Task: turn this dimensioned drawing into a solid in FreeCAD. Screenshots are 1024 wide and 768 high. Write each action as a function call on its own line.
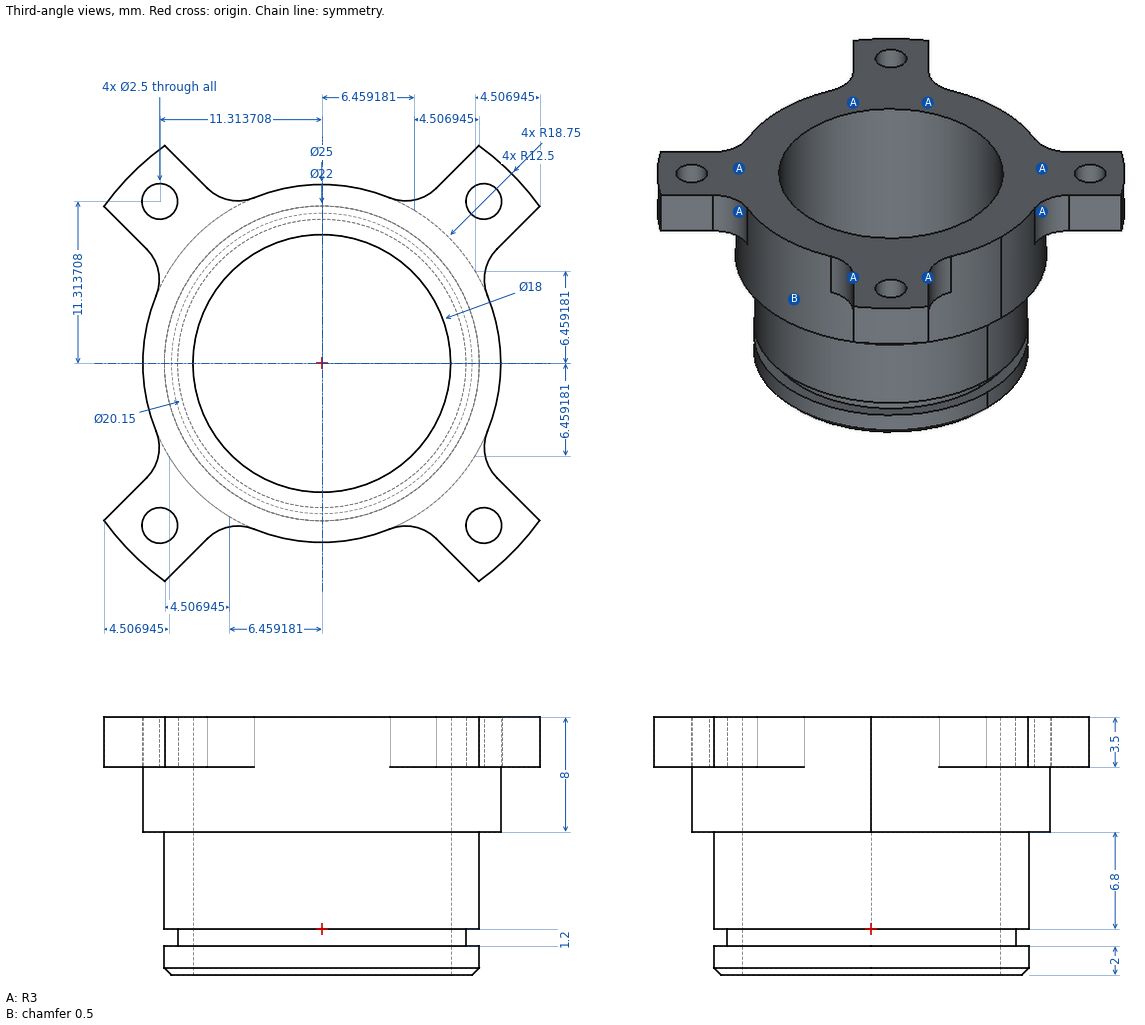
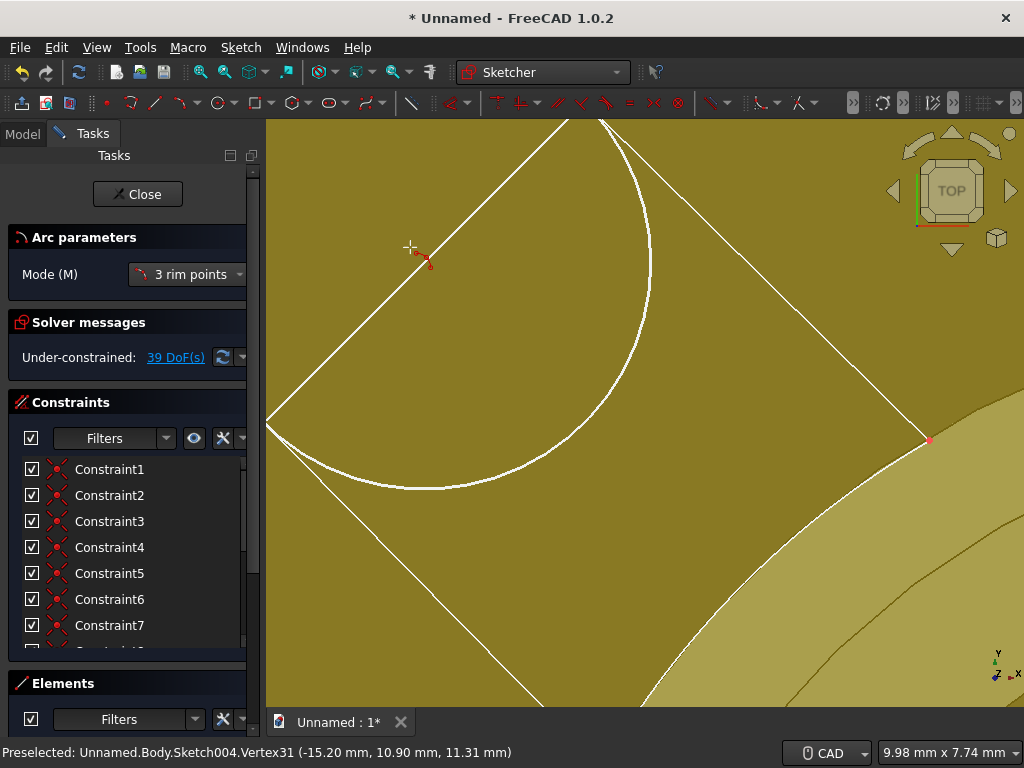
click(411, 243)
key(Escape)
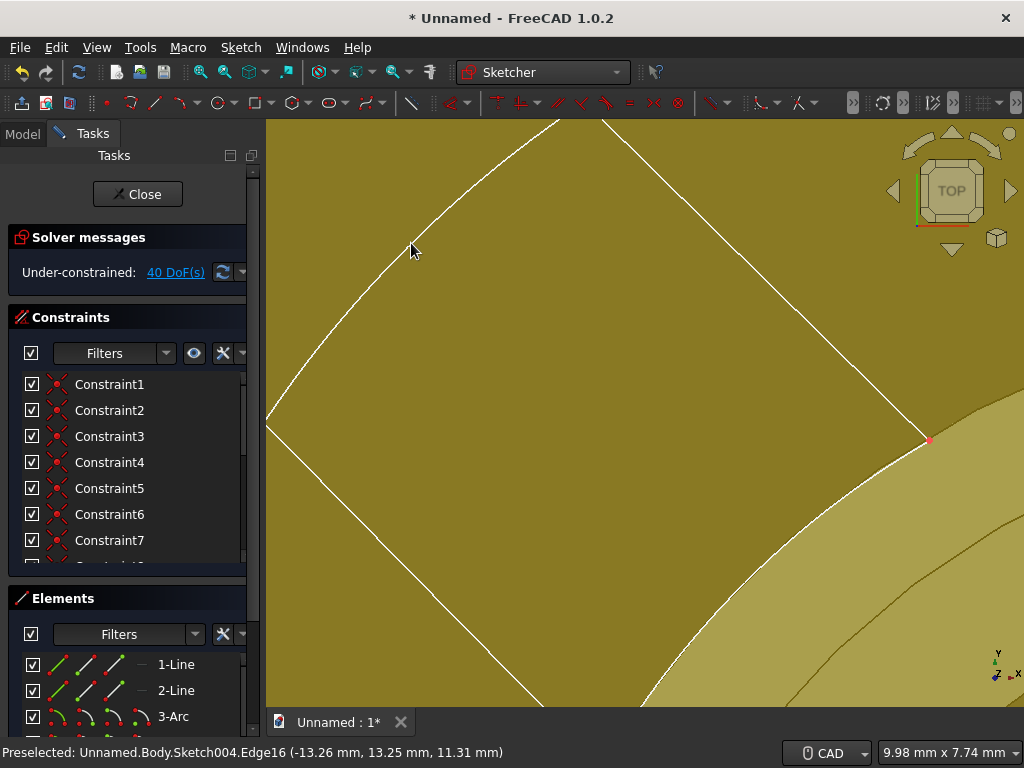
scroll(410, 247, down, 9)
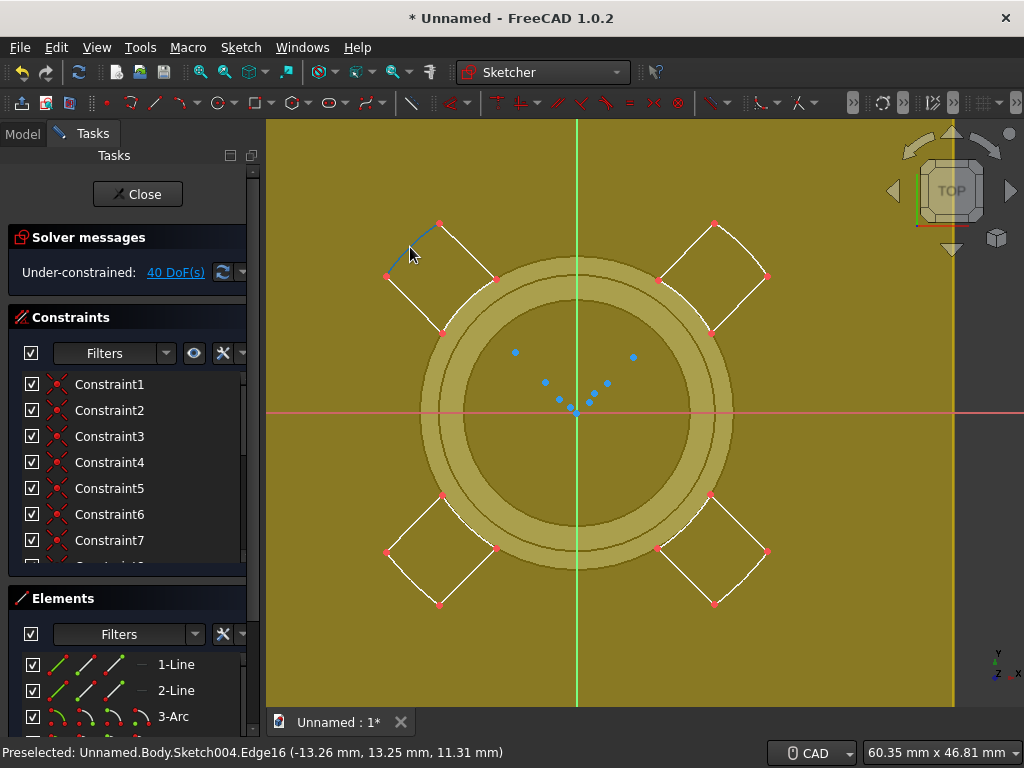
click(699, 314)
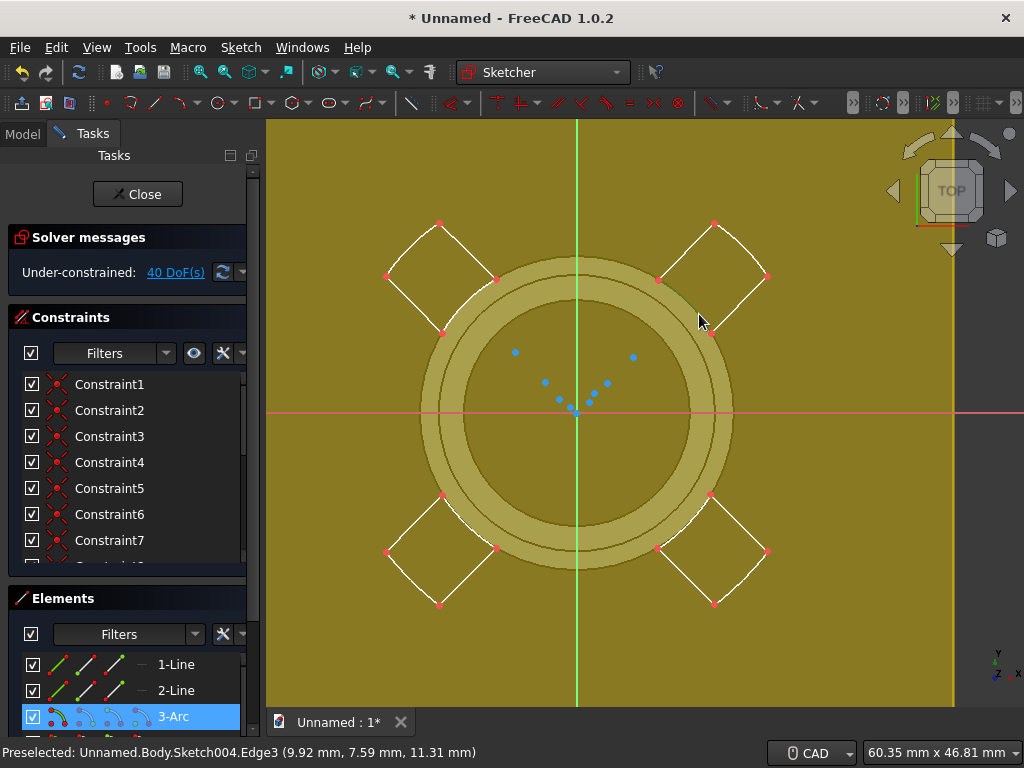
click(754, 258)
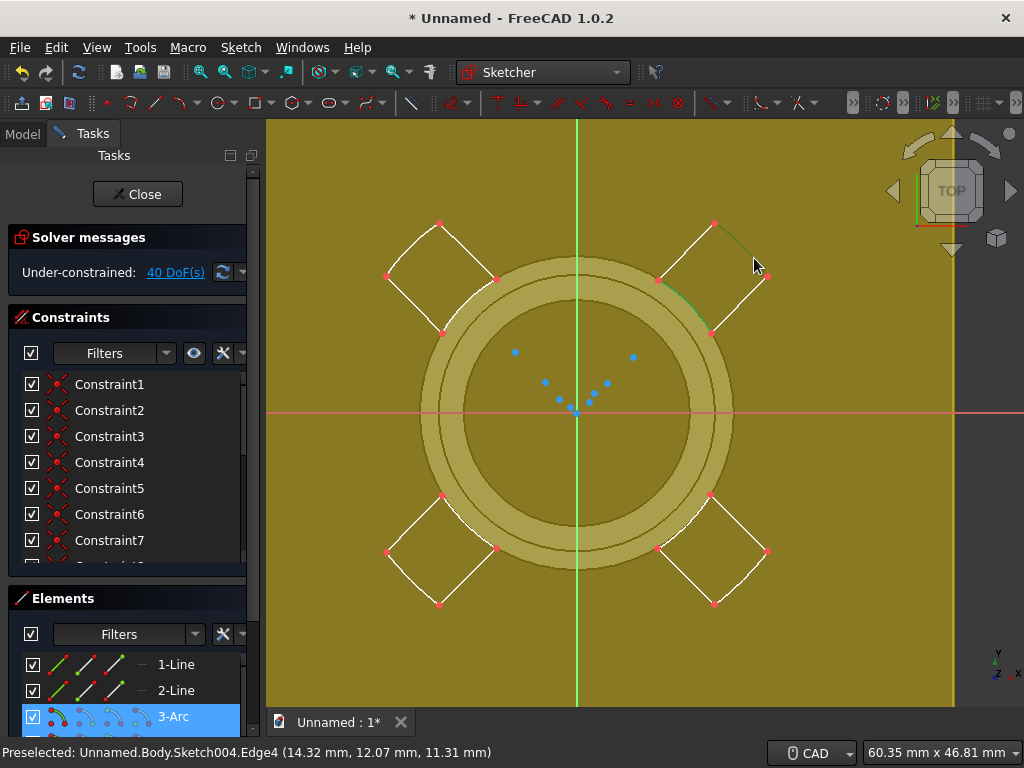
click(498, 104)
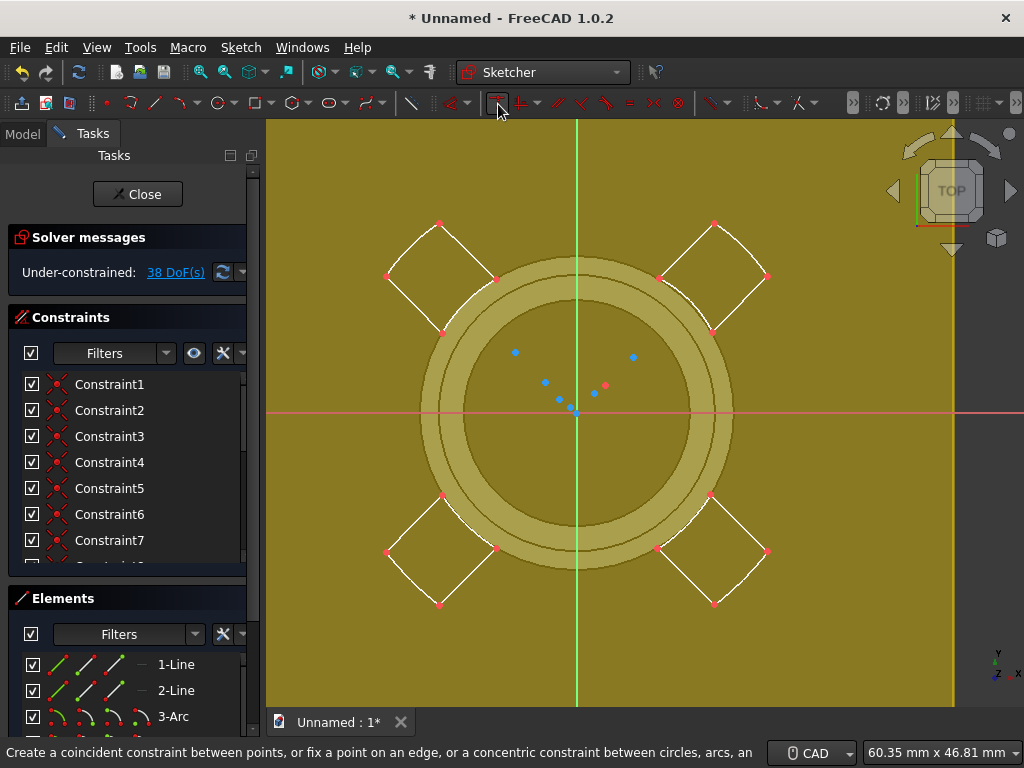
click(700, 313)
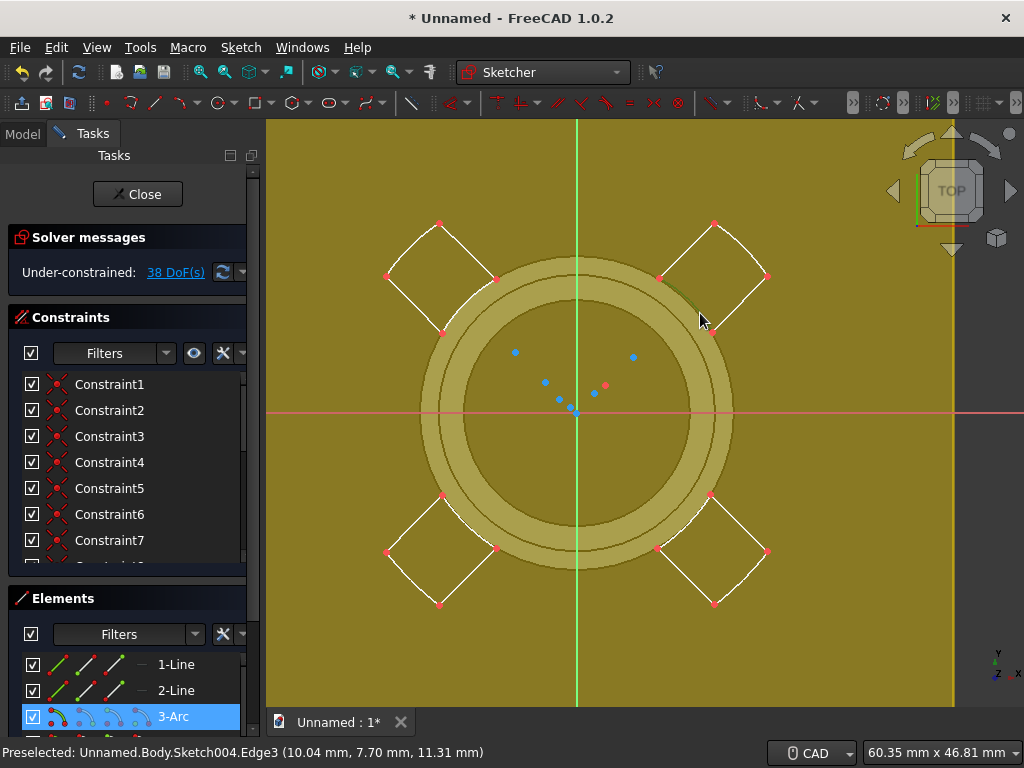
click(676, 535)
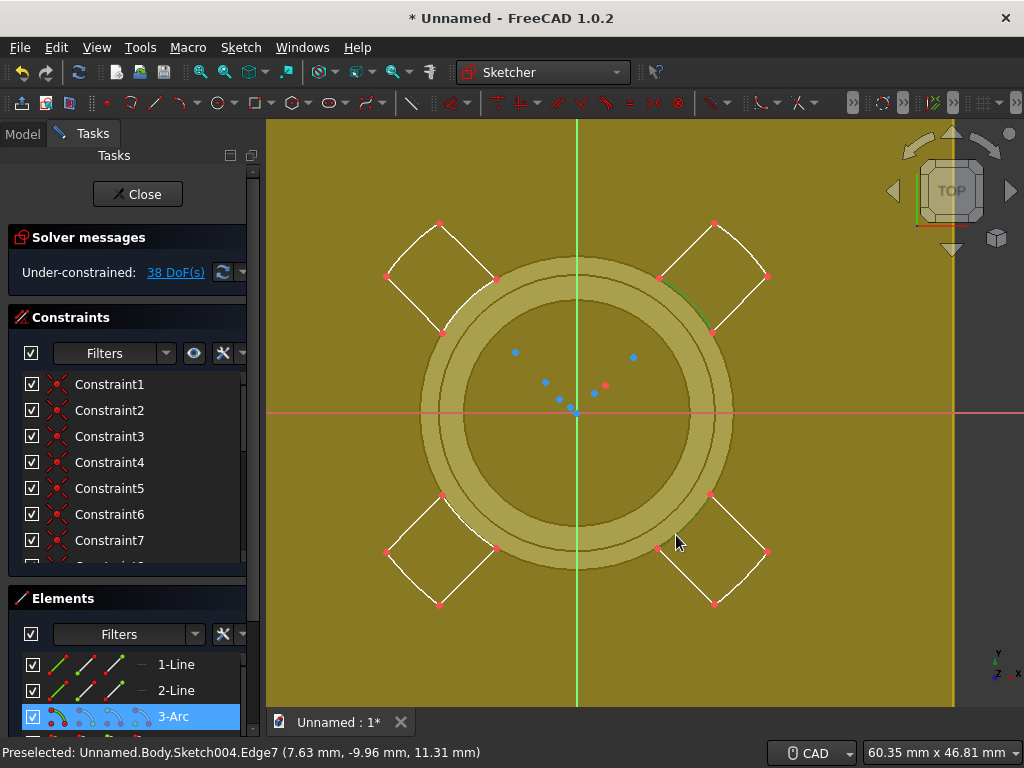
click(498, 104)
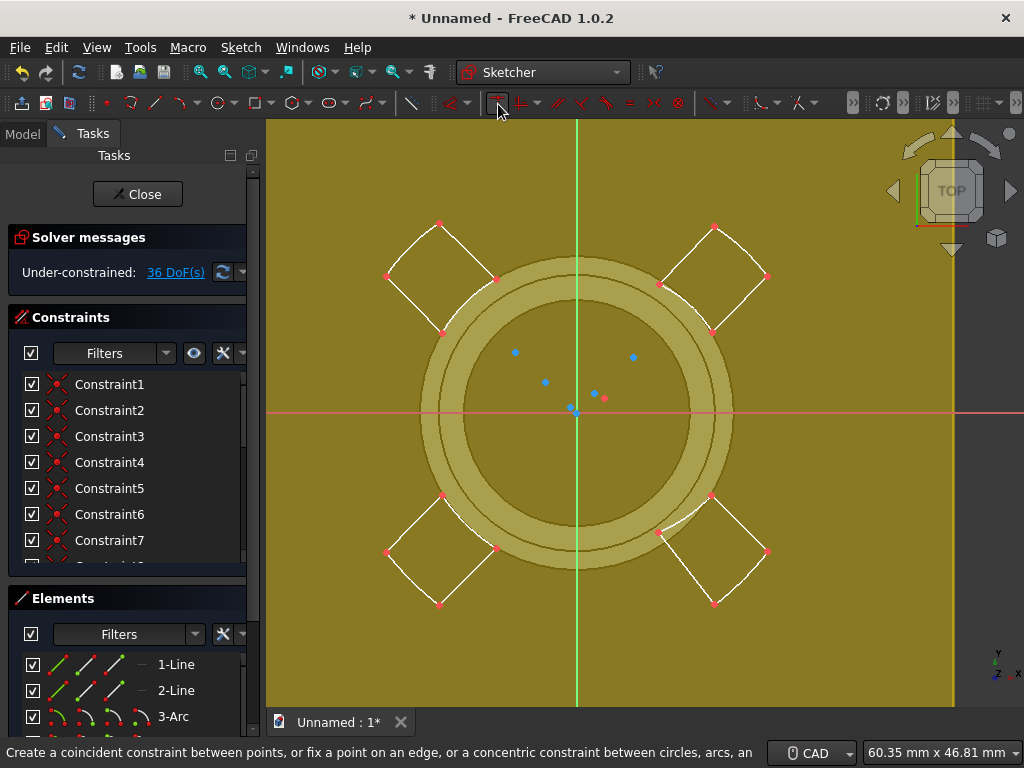
click(699, 315)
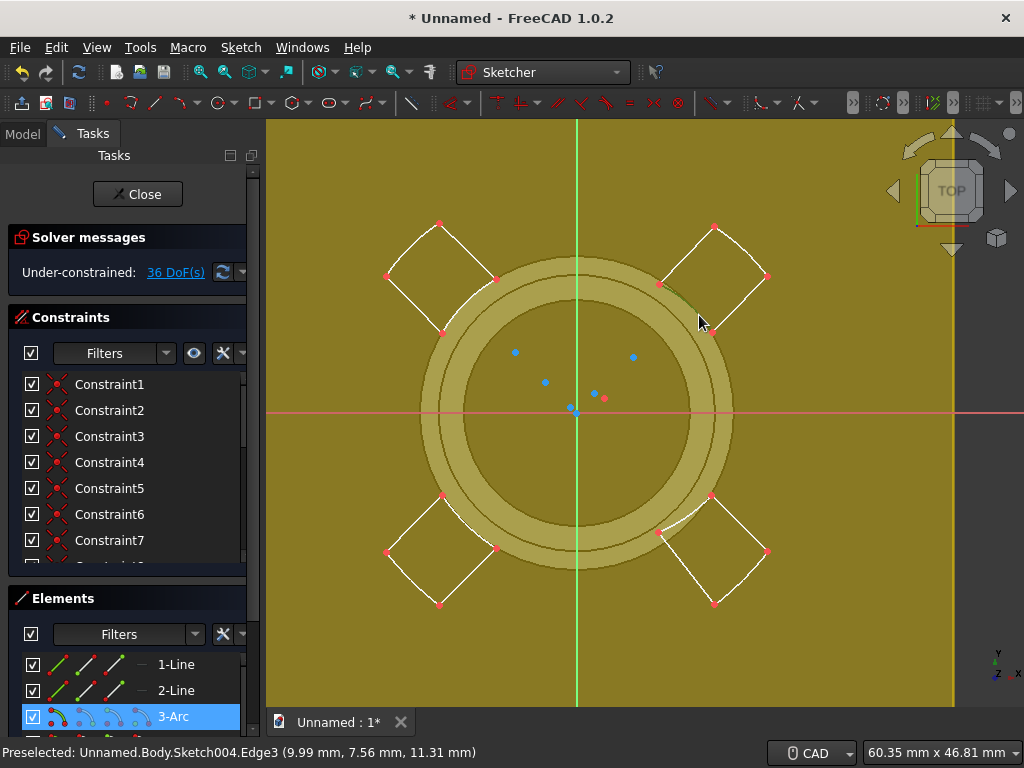
click(732, 590)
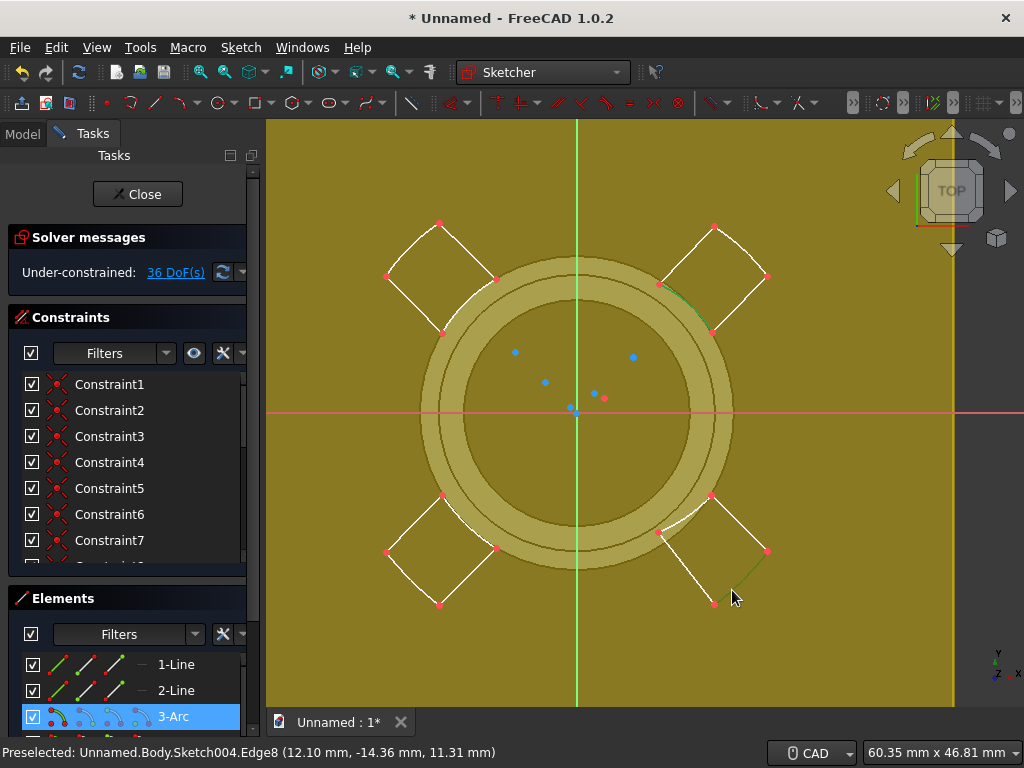
click(498, 104)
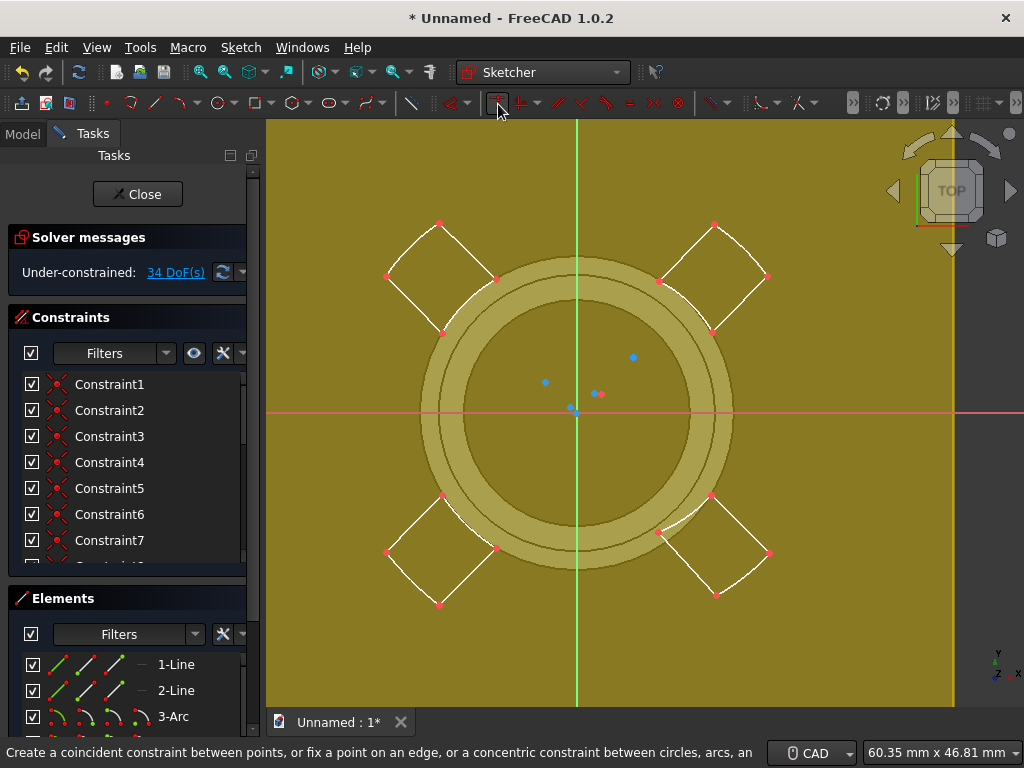
click(700, 314)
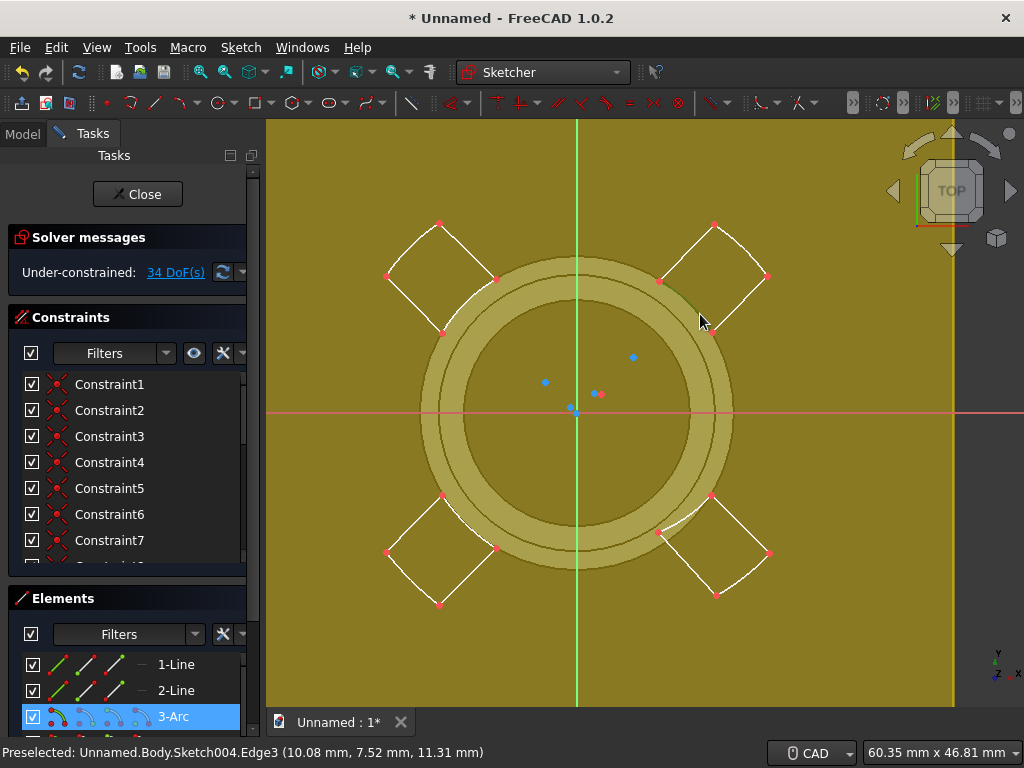
click(456, 513)